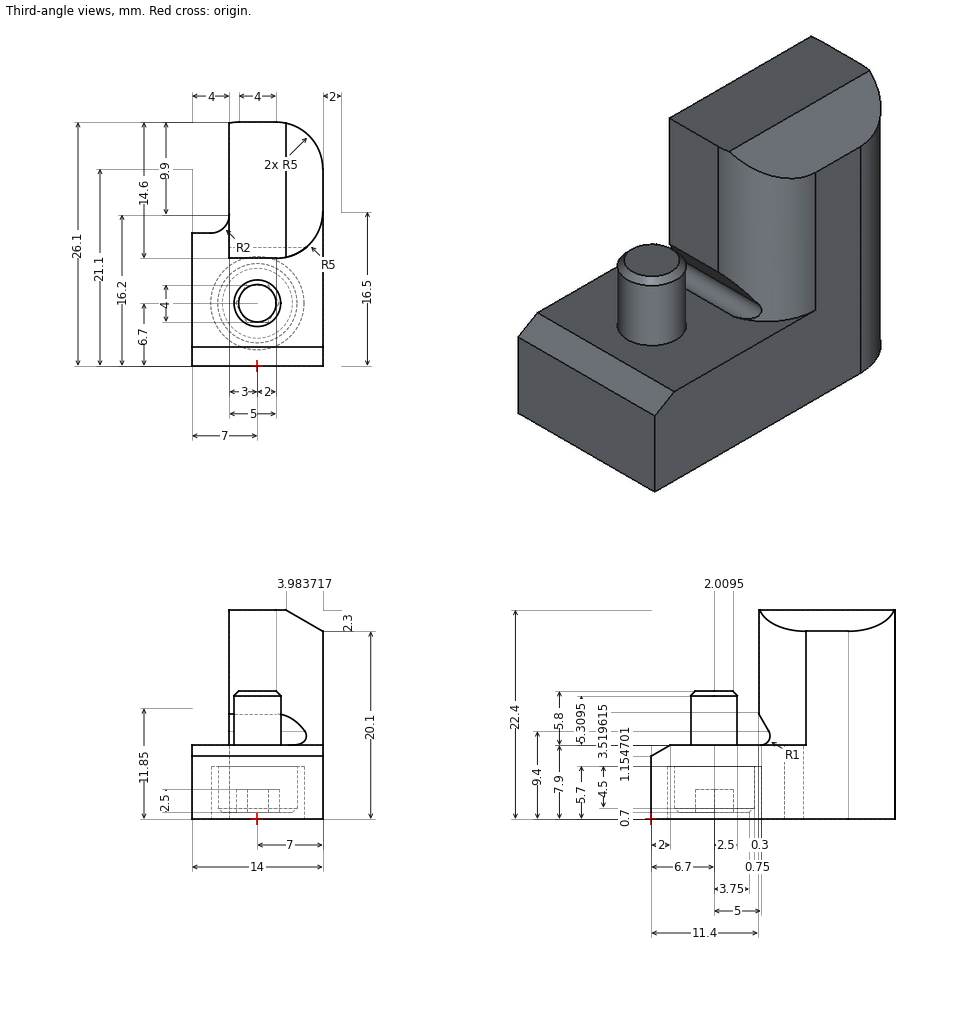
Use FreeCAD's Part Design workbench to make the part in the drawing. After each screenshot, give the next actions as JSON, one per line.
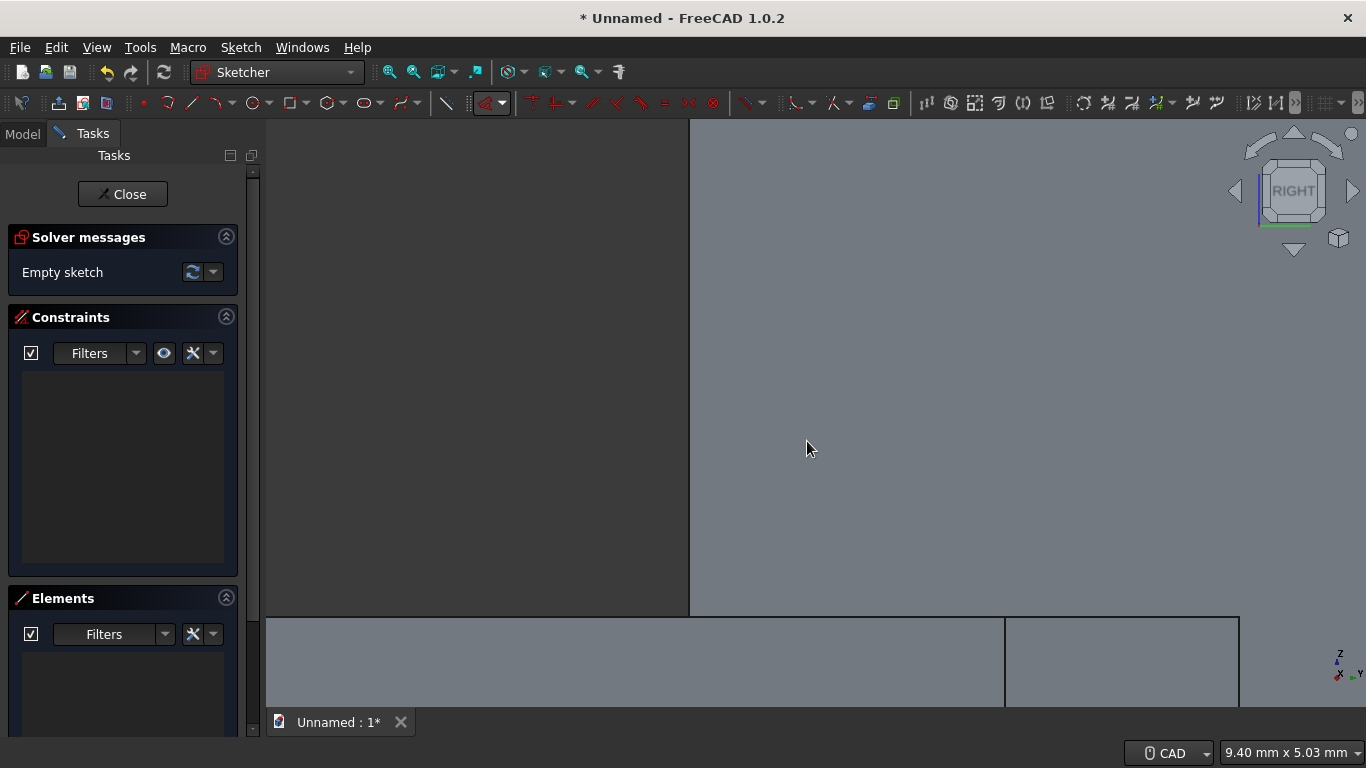
{"action": "left_click", "coordinate": [168, 104]}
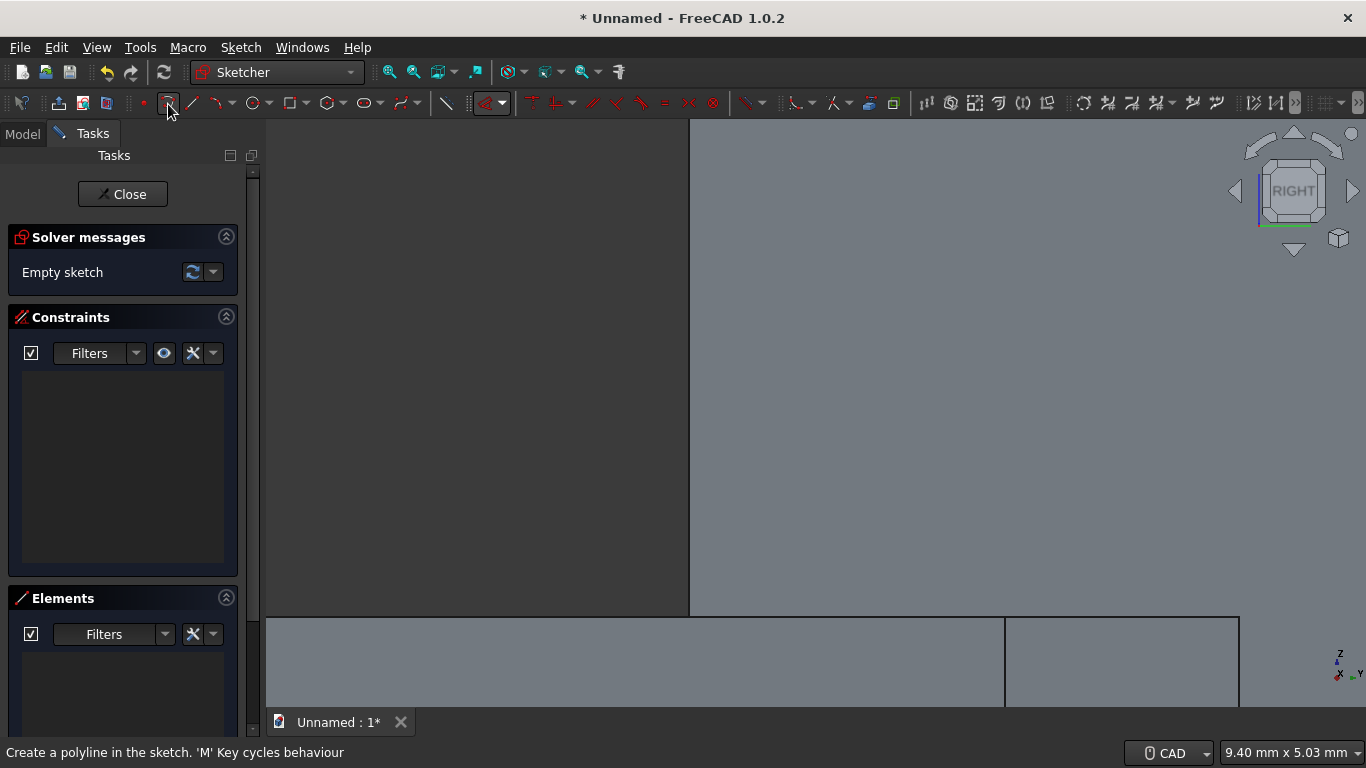
{"action": "left_click", "coordinate": [814, 441]}
{"action": "left_click", "coordinate": [677, 205]}
{"action": "left_click", "coordinate": [677, 617]}
{"action": "left_click", "coordinate": [712, 617]}
{"action": "right_click", "coordinate": [712, 617]}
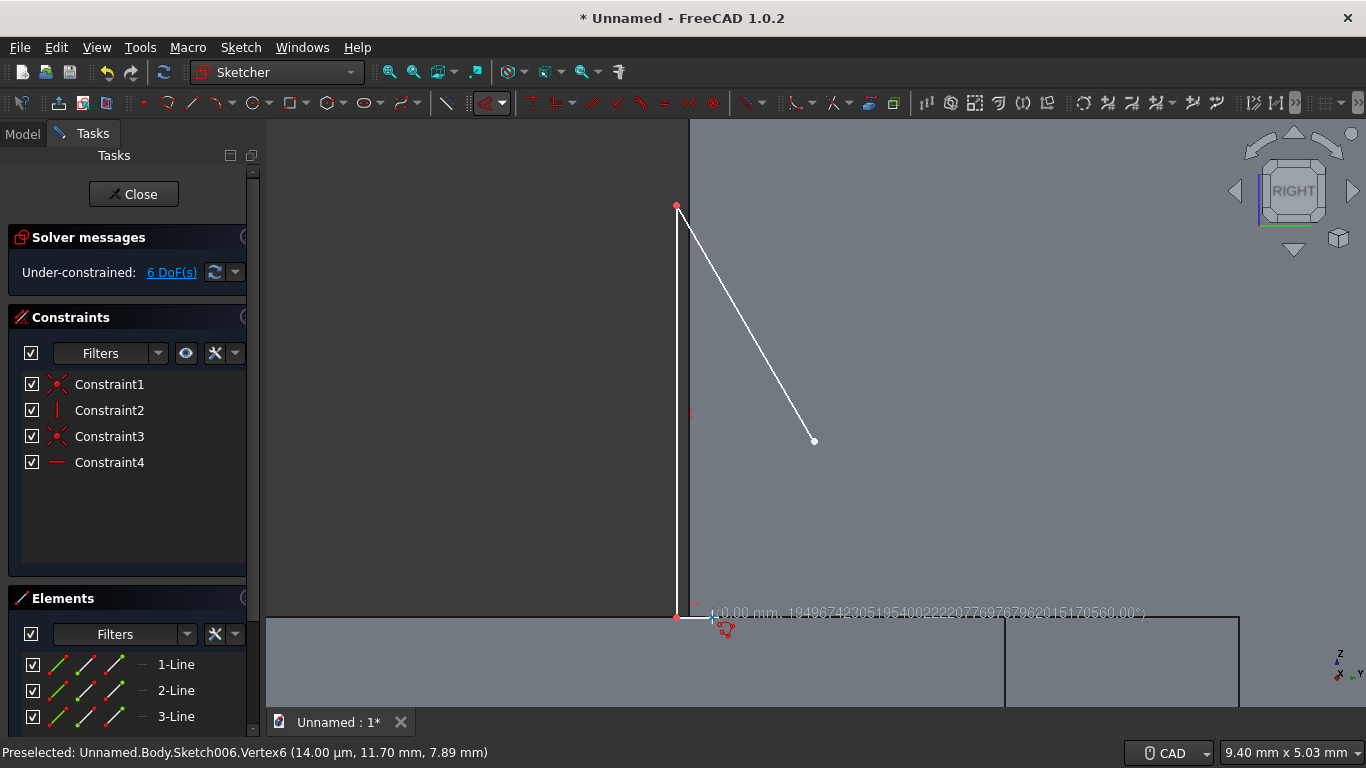
{"action": "left_click", "coordinate": [216, 104]}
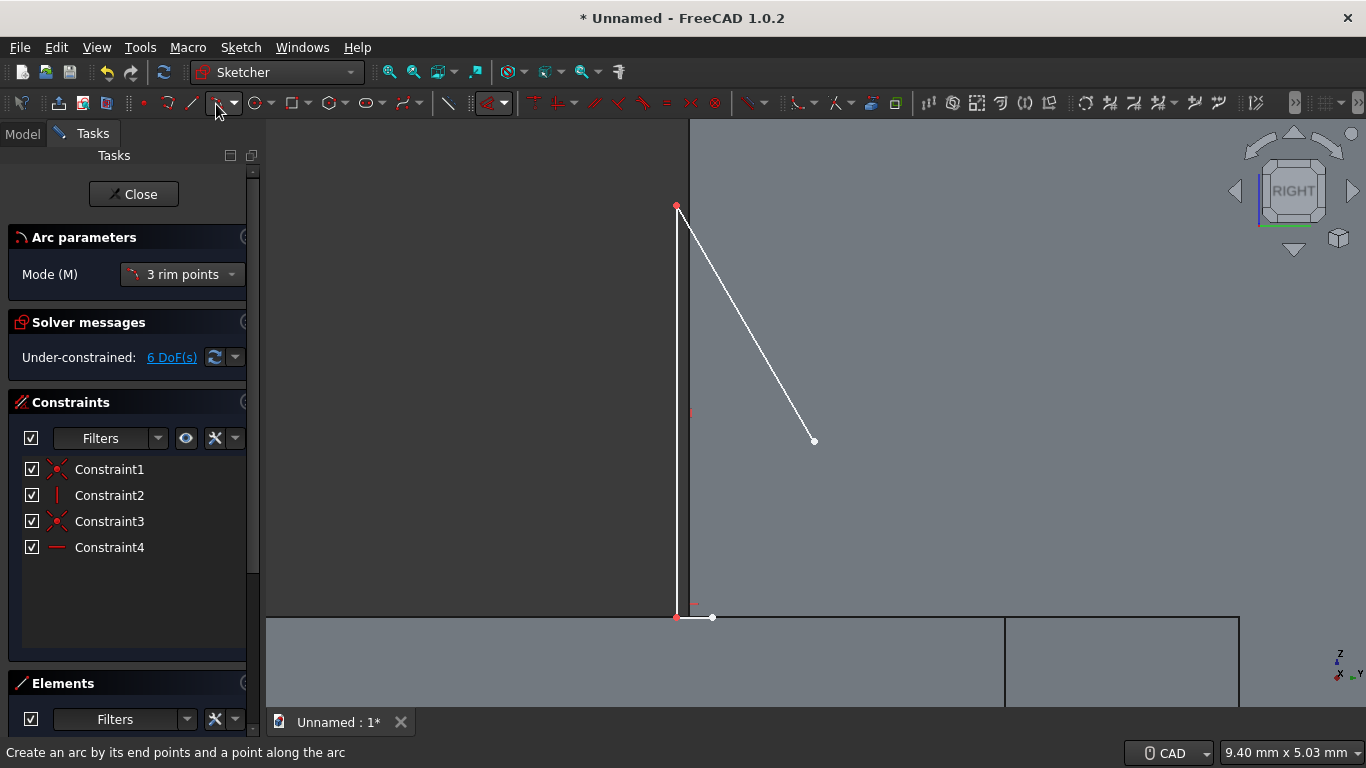
{"action": "left_click", "coordinate": [712, 618]}
{"action": "left_click", "coordinate": [814, 442]}
{"action": "left_click", "coordinate": [814, 558]}
{"action": "key", "text": "Escape"}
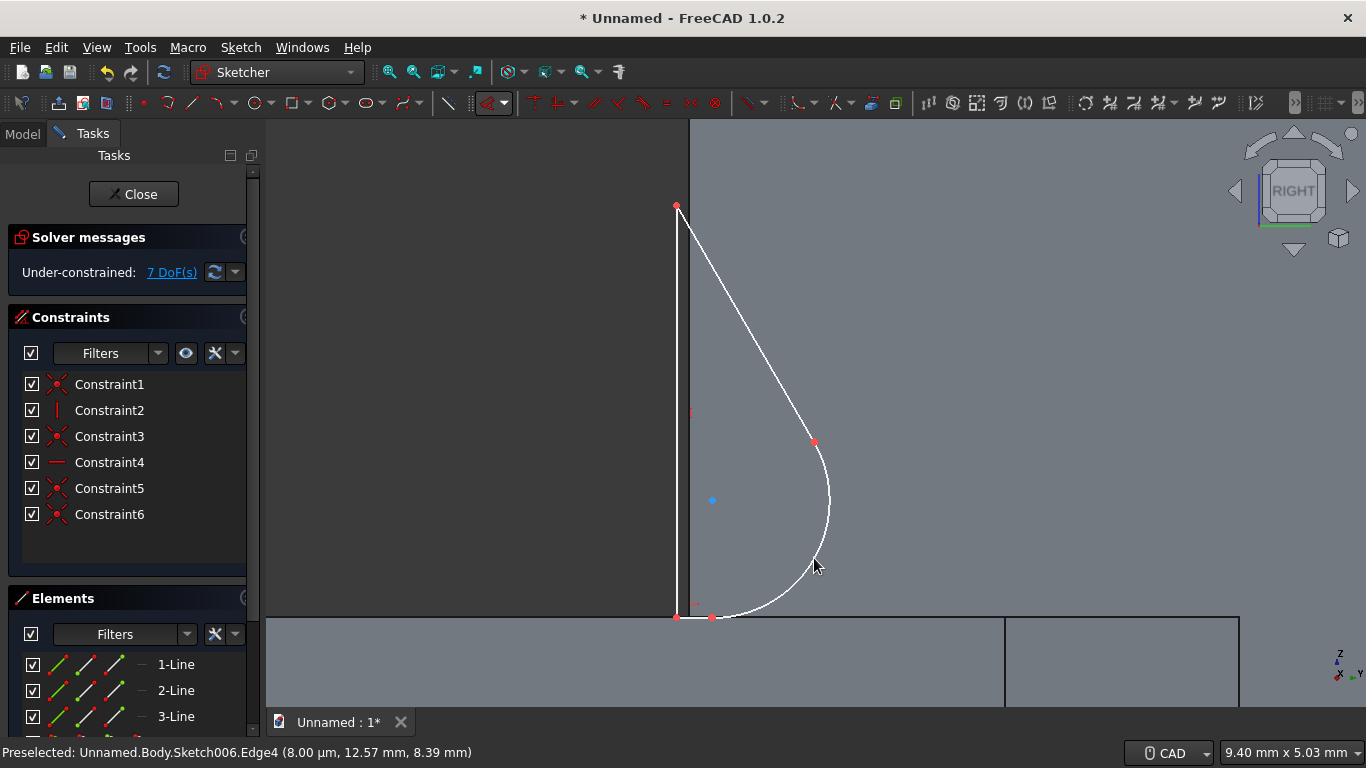
{"action": "left_click", "coordinate": [773, 371]}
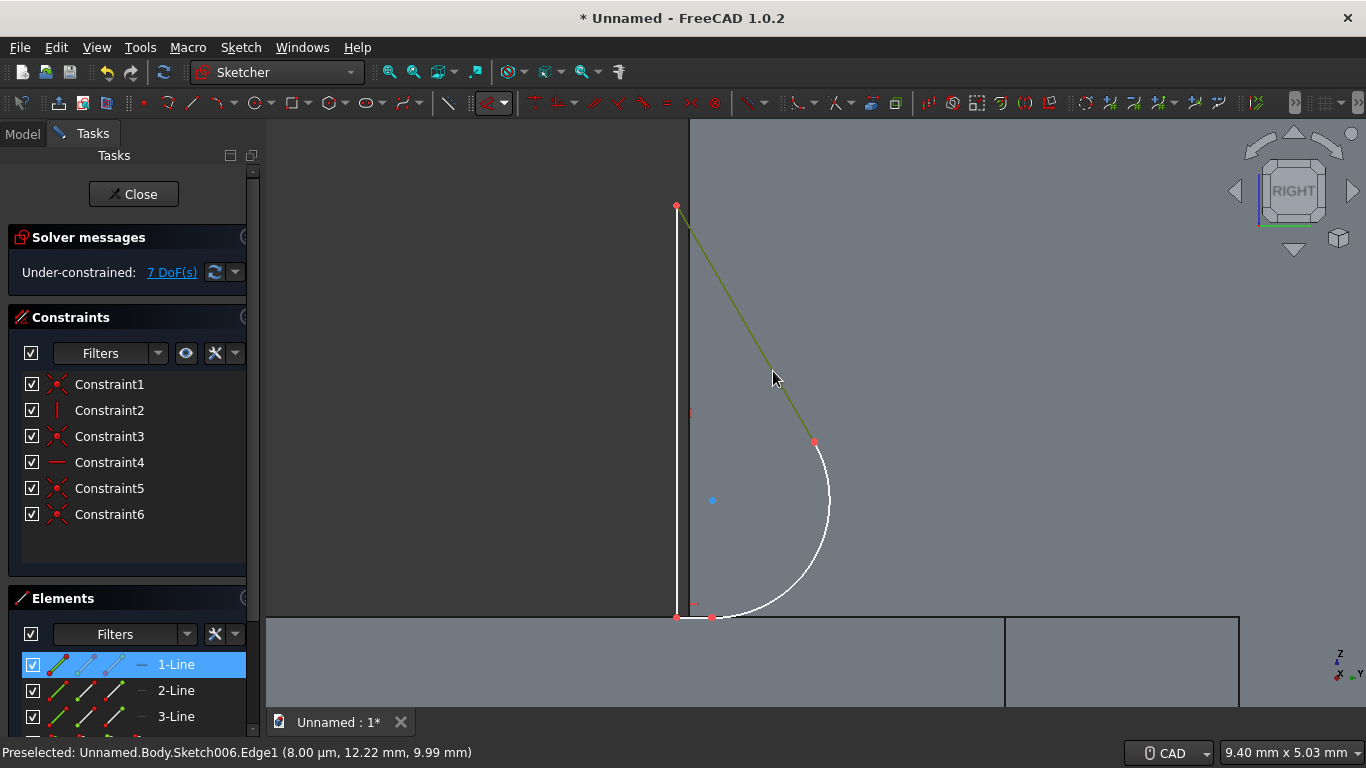
{"action": "left_click", "coordinate": [781, 596]}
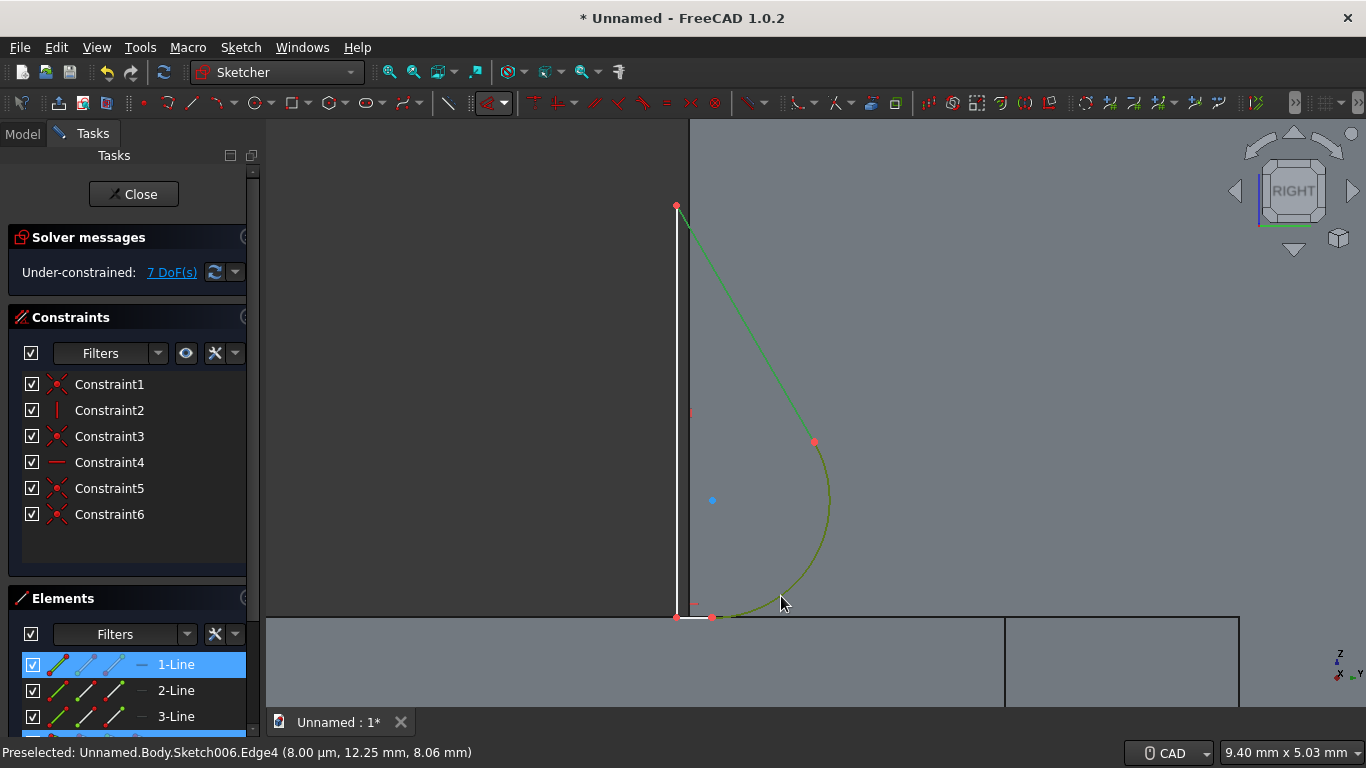
{"action": "left_click", "coordinate": [644, 104]}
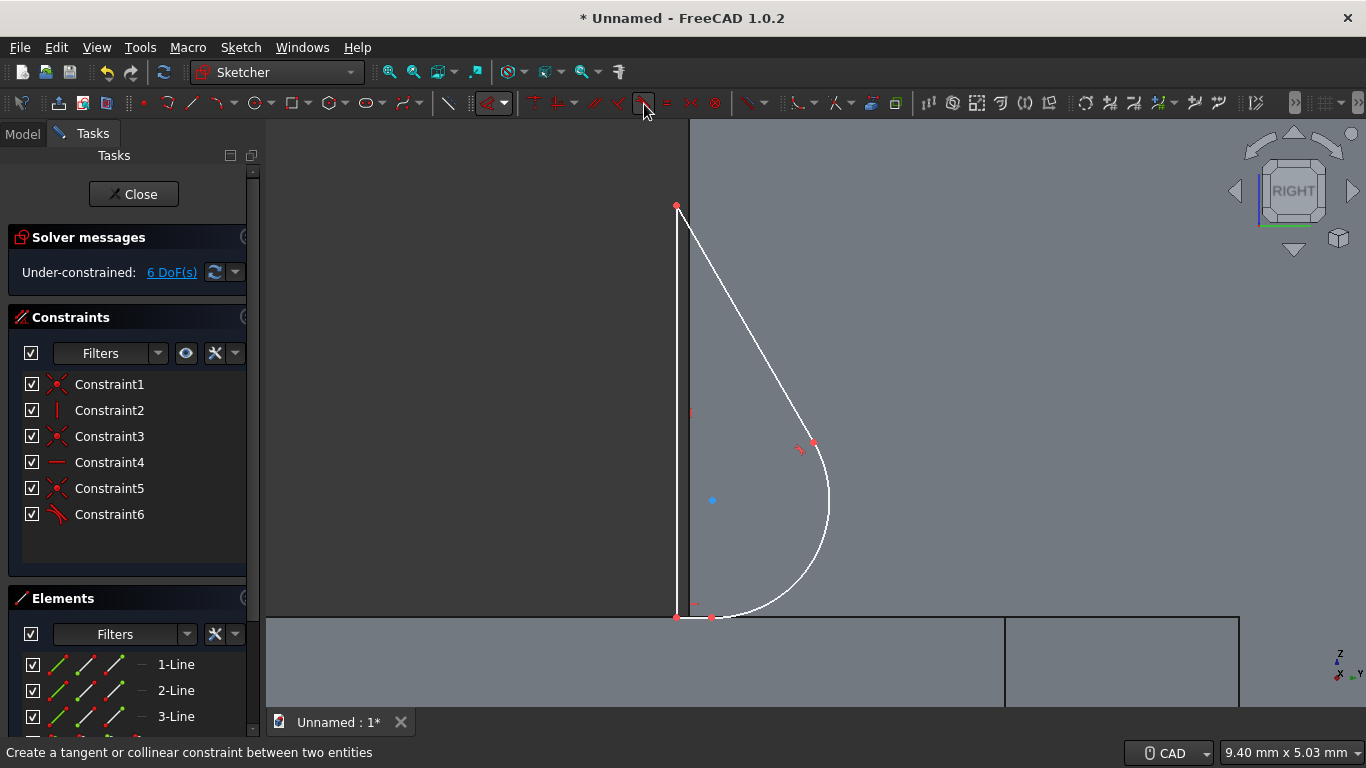
{"action": "scroll", "coordinate": [687, 618], "scroll_direction": "up", "scroll_amount": 2}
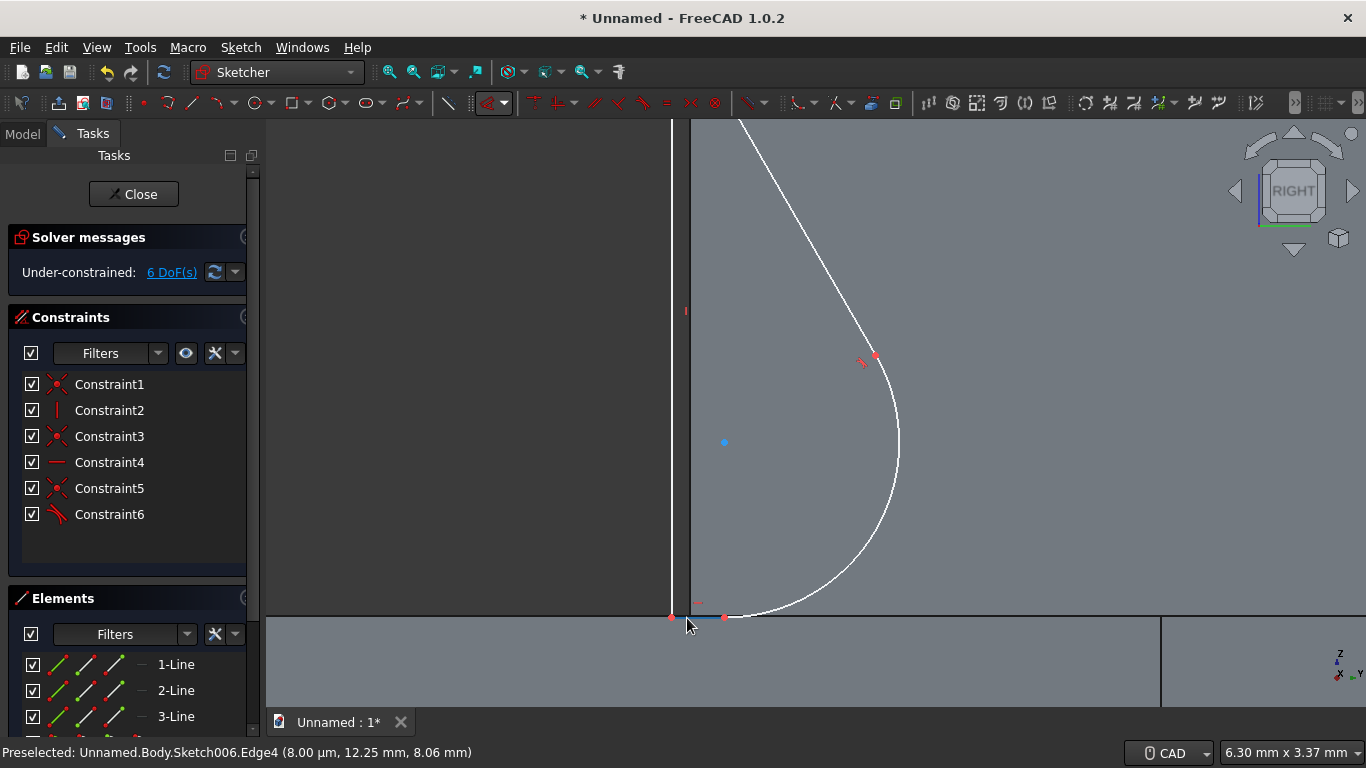
{"action": "left_click", "coordinate": [688, 618]}